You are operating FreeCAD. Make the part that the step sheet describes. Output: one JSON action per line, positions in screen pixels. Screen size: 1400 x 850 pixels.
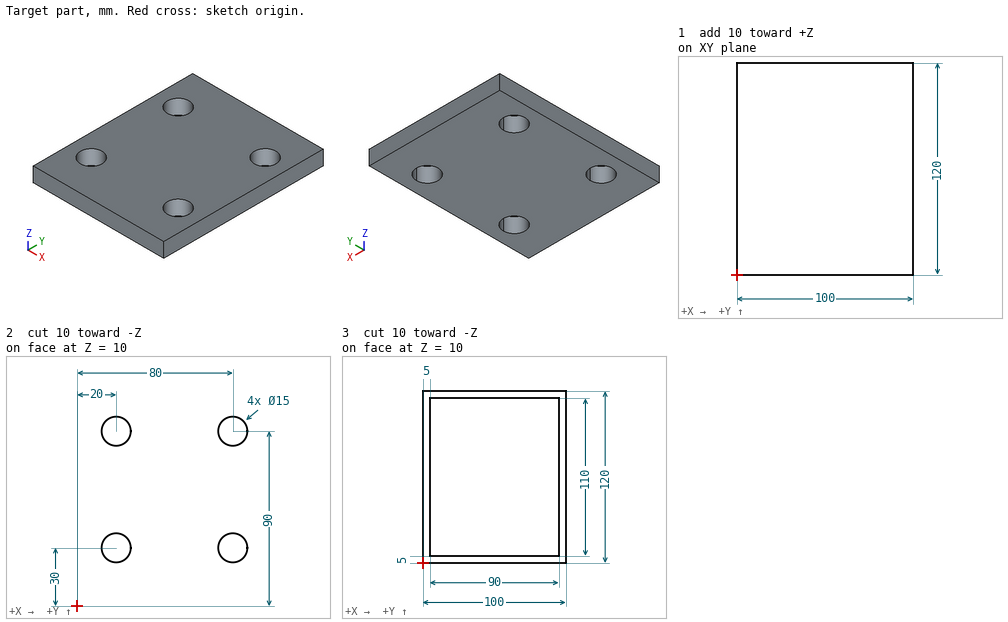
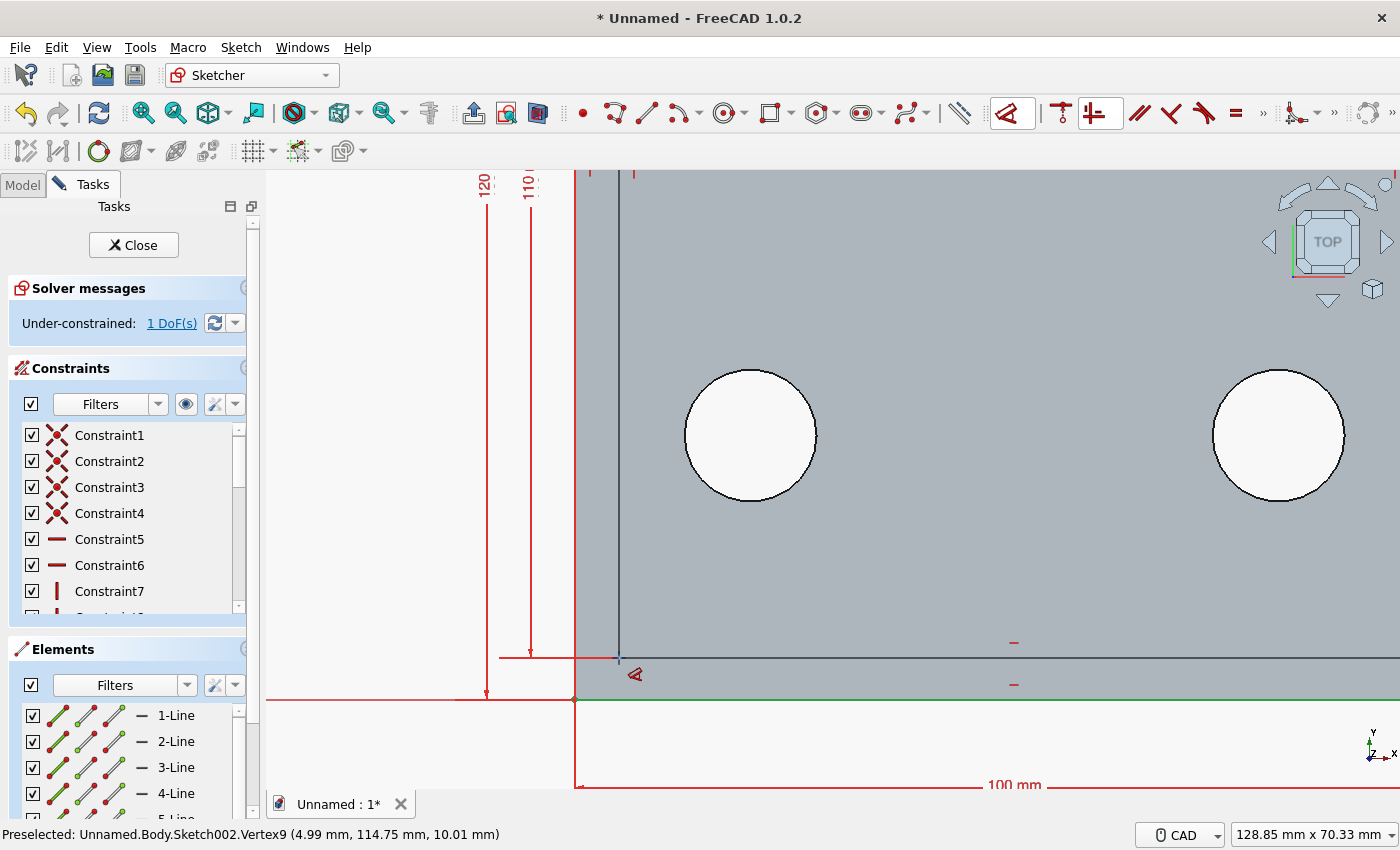
{"action": "left_click", "coordinate": [619, 658]}
{"action": "left_click", "coordinate": [541, 679]}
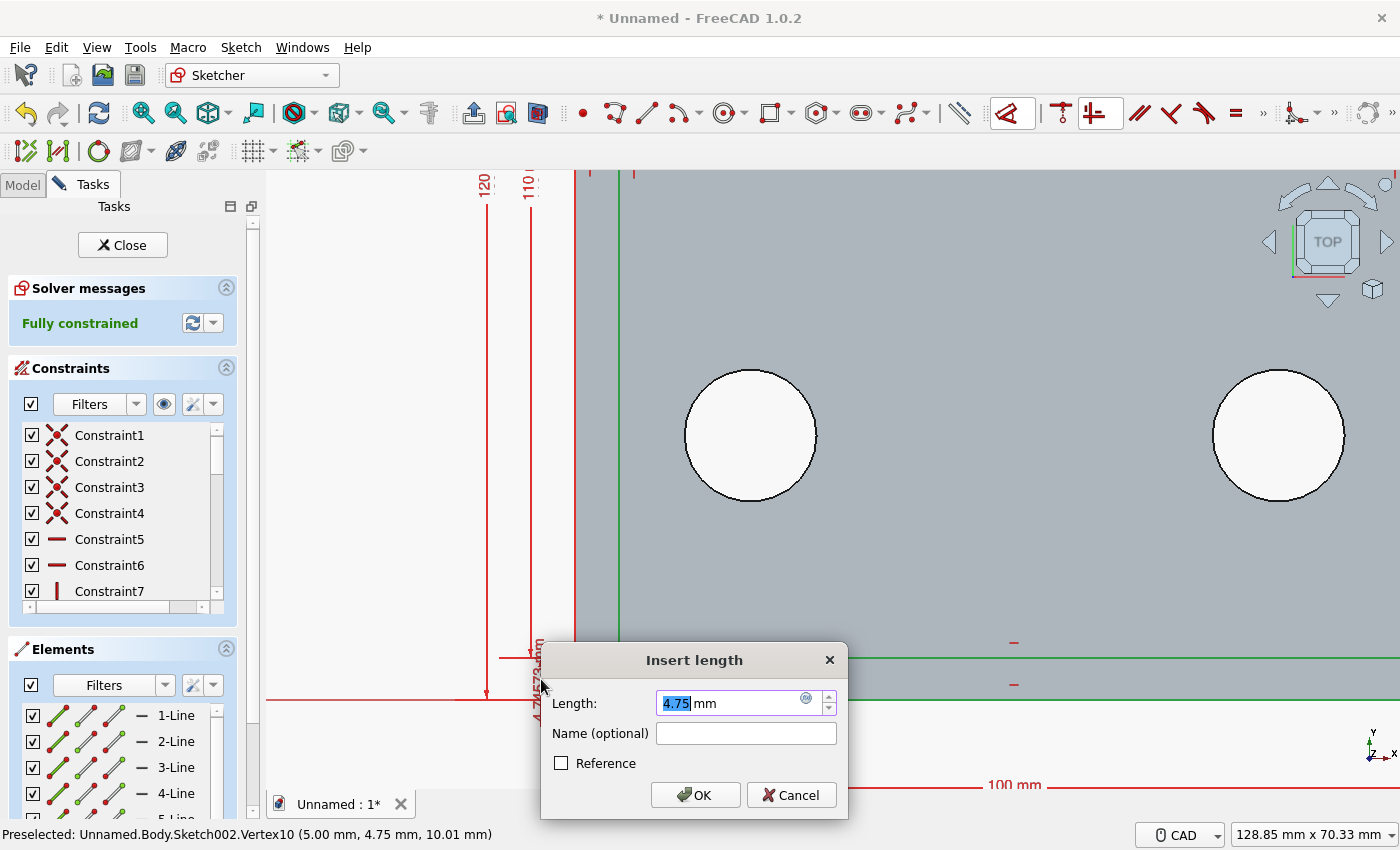
{"action": "type", "text": "5"}
{"action": "key", "text": "Return"}
{"action": "key", "text": "Escape"}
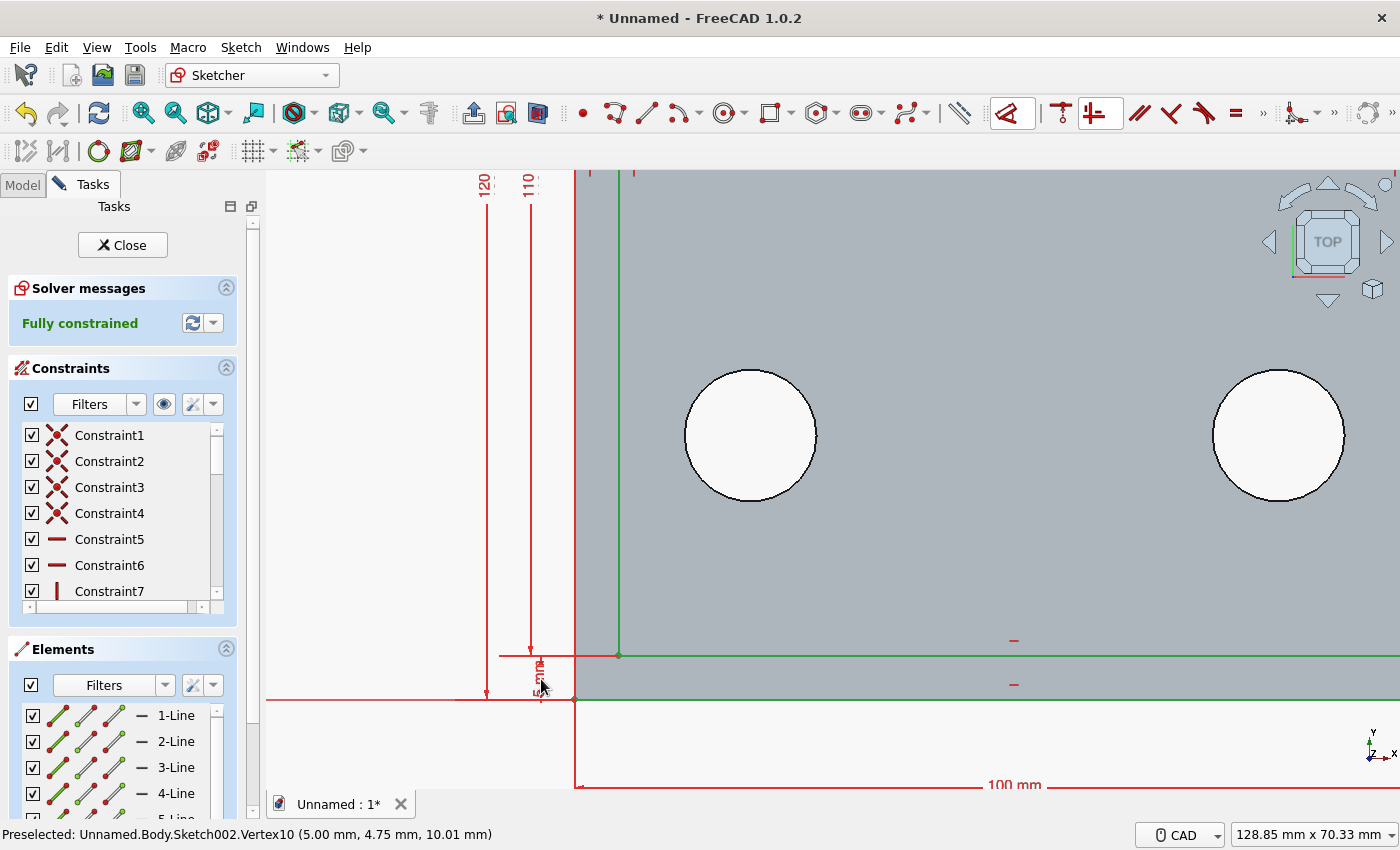
{"action": "left_click", "coordinate": [123, 245]}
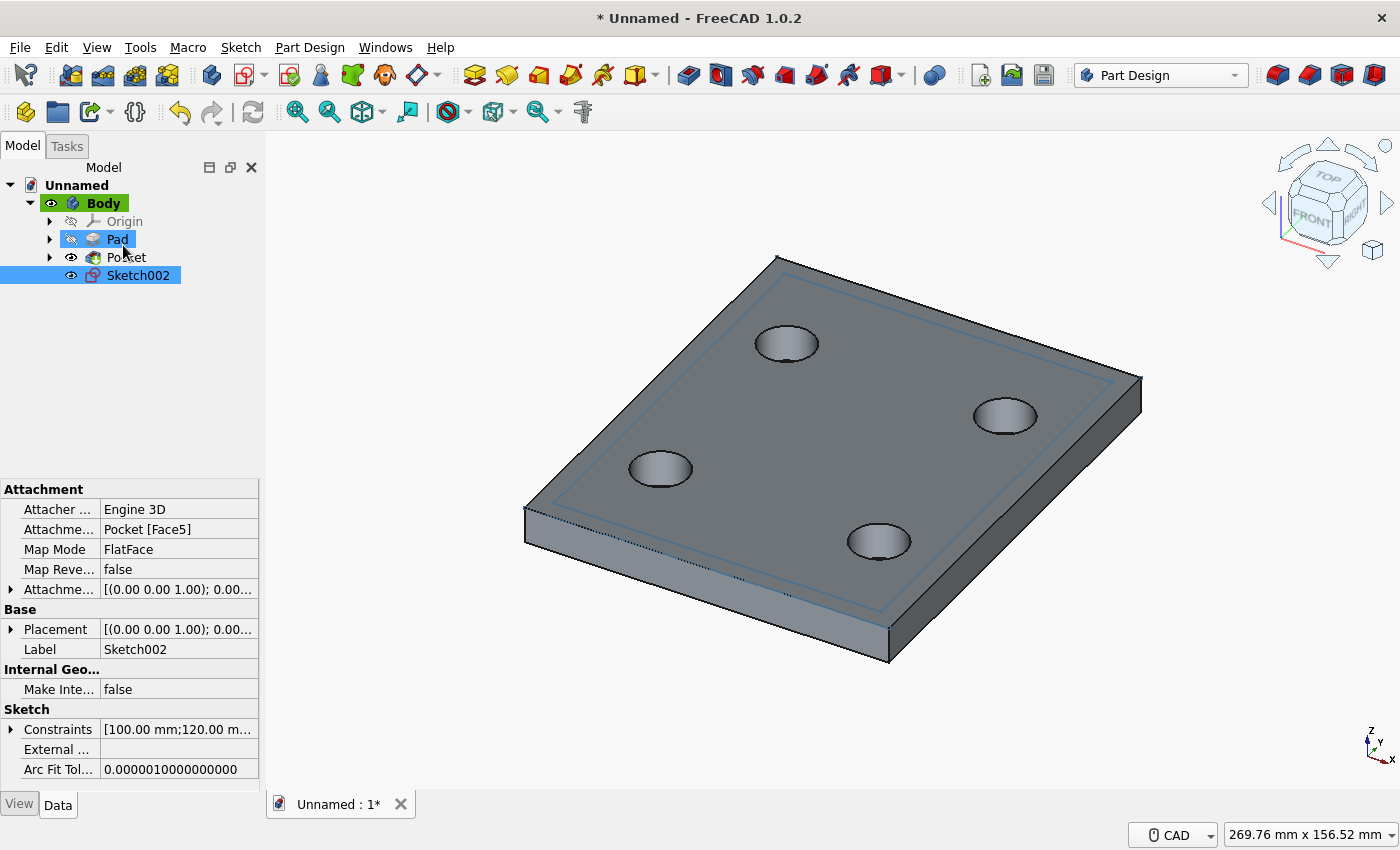
{"action": "left_click", "coordinate": [690, 76]}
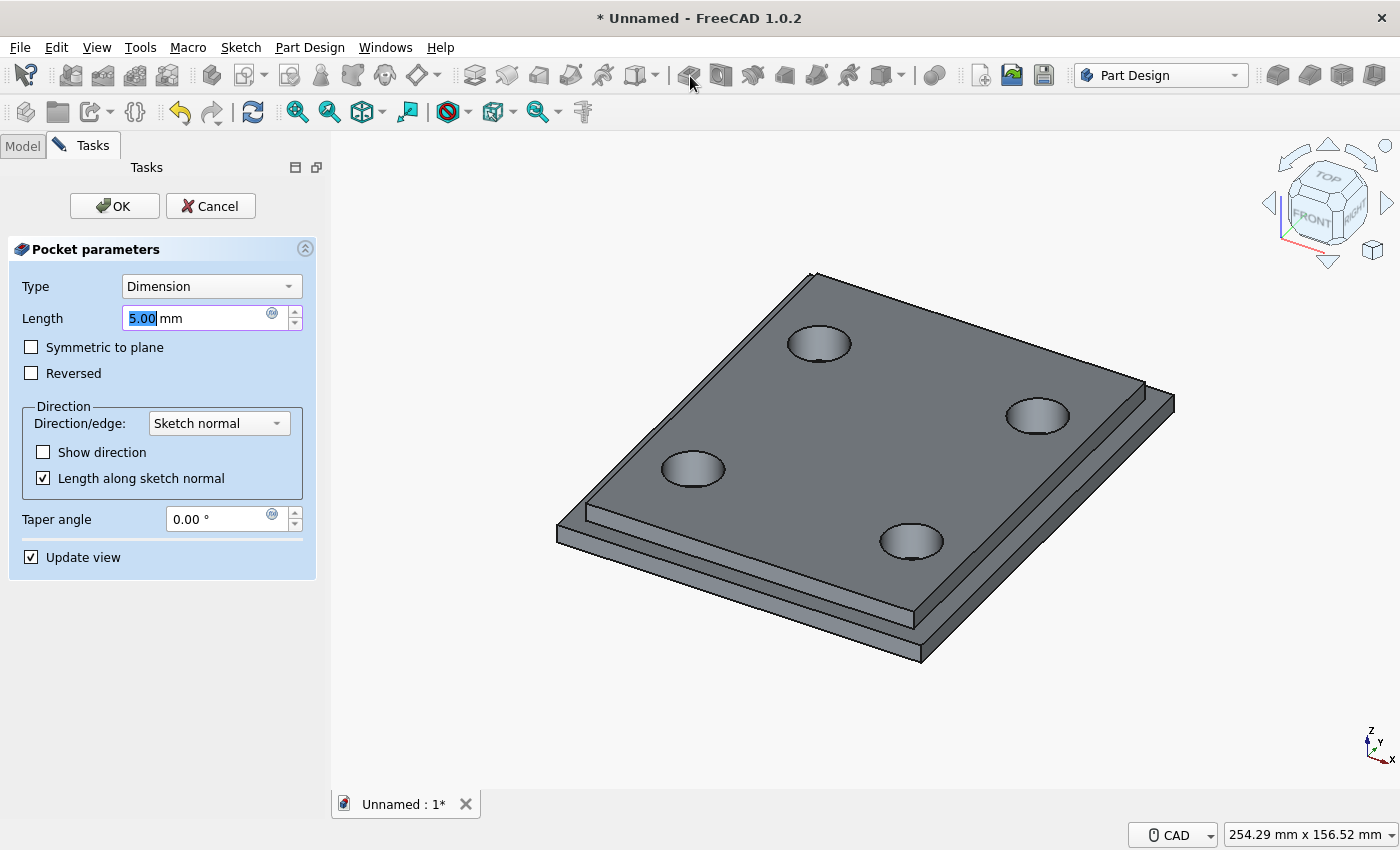
{"action": "type", "text": "10"}
{"action": "key", "text": "Tab"}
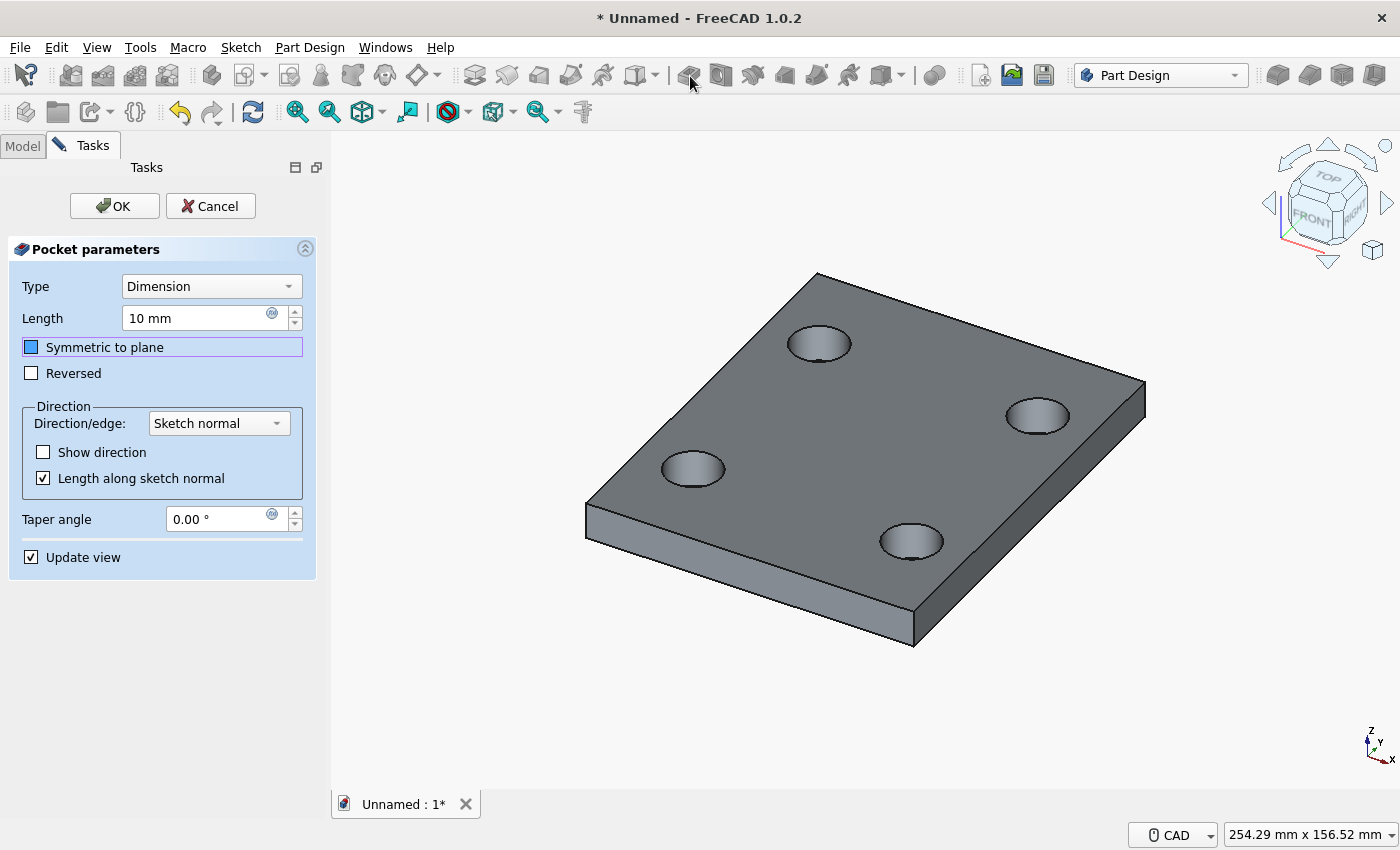
{"action": "left_click", "coordinate": [115, 206]}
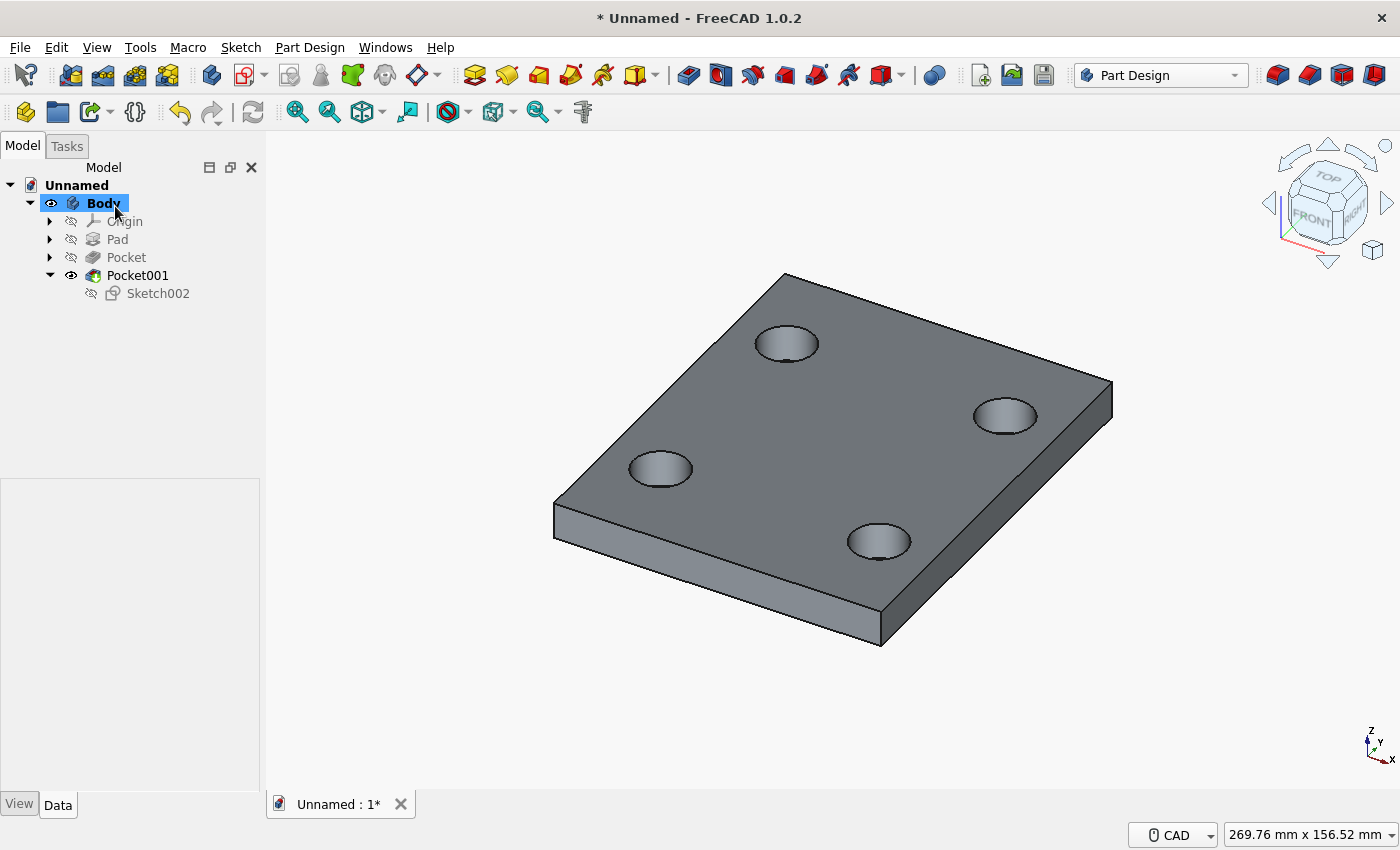
{"action": "key", "text": "0"}